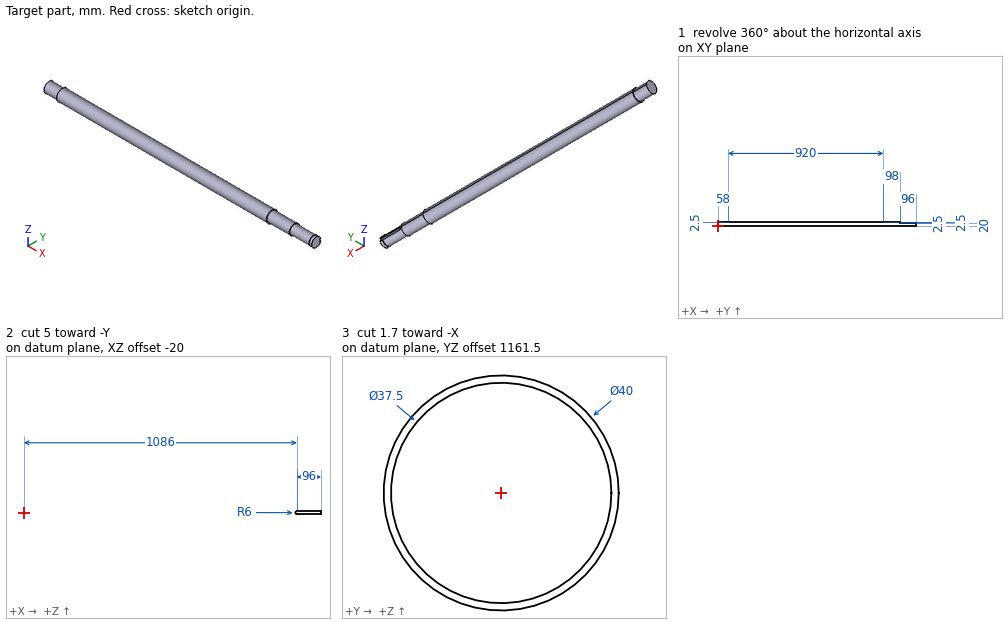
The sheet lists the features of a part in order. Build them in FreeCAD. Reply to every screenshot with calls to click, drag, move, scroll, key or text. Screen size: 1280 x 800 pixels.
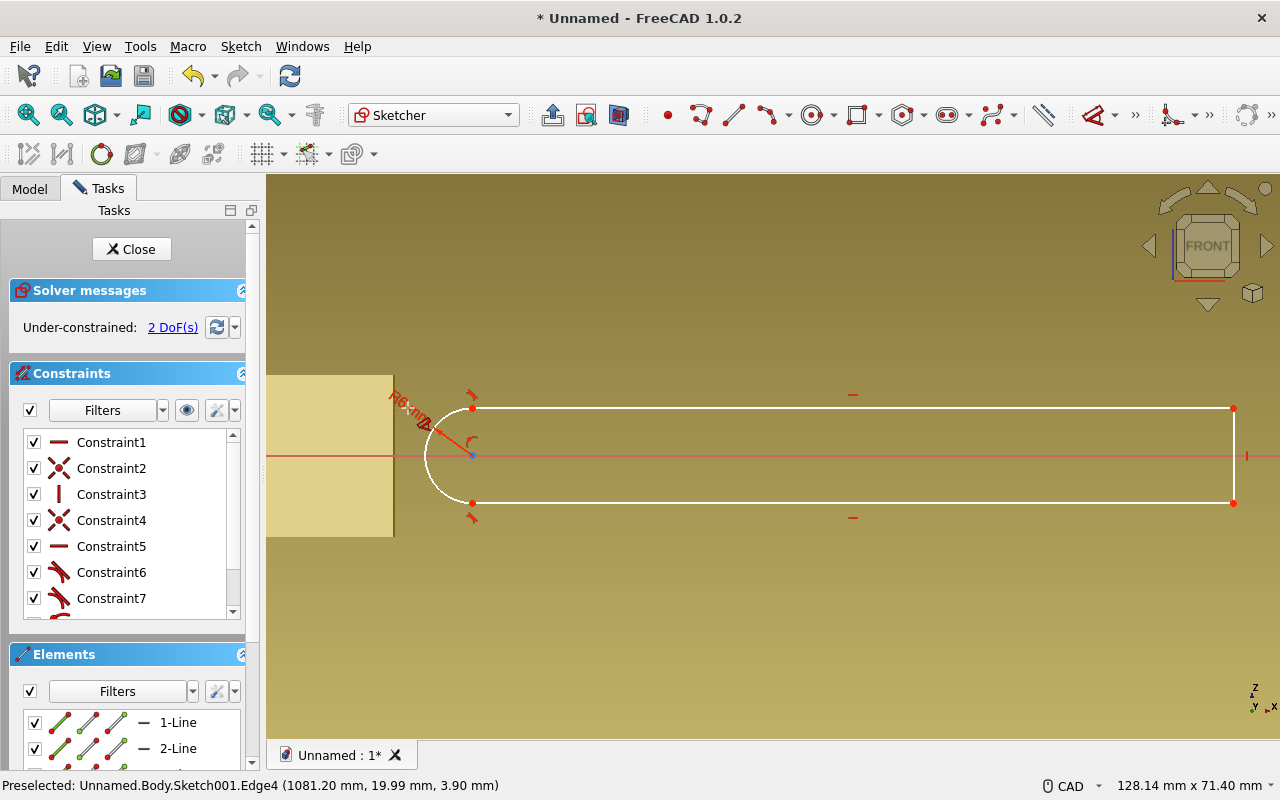
click(701, 408)
click(794, 374)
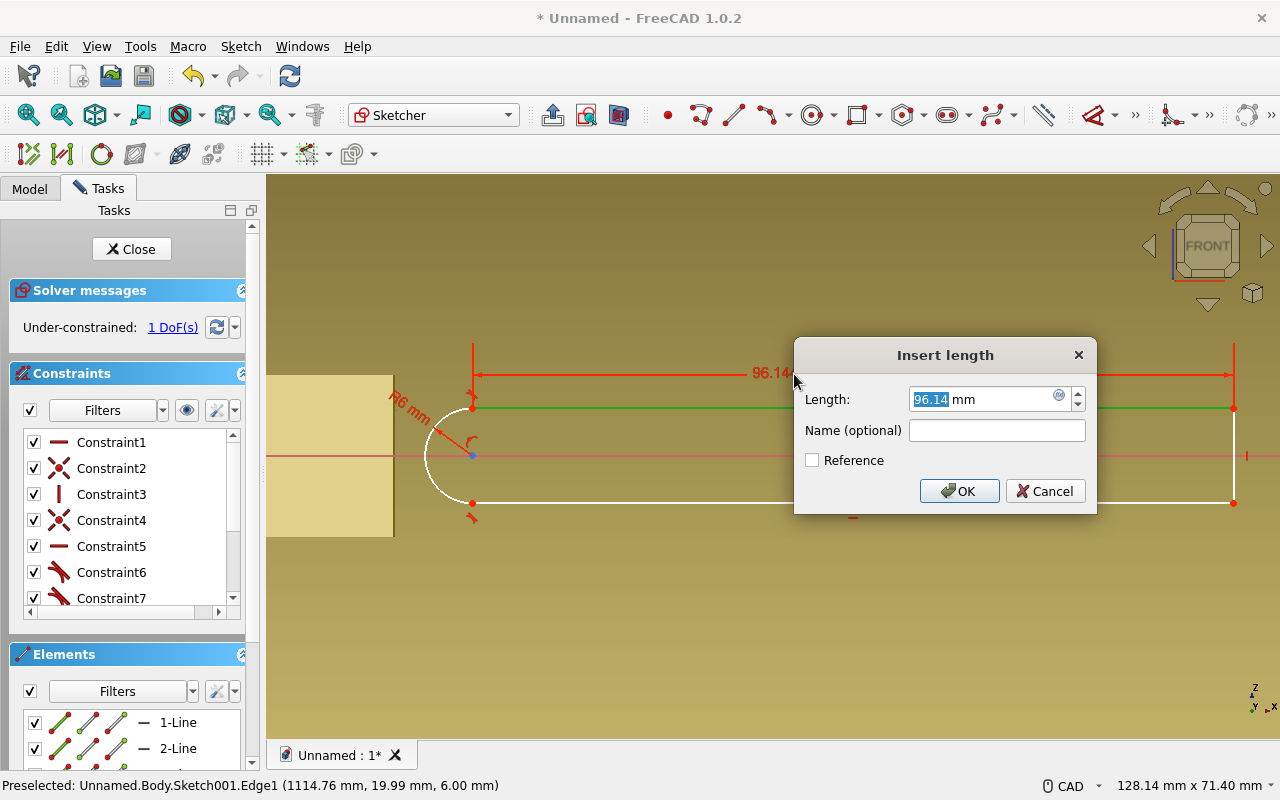
text(96)
key(Return)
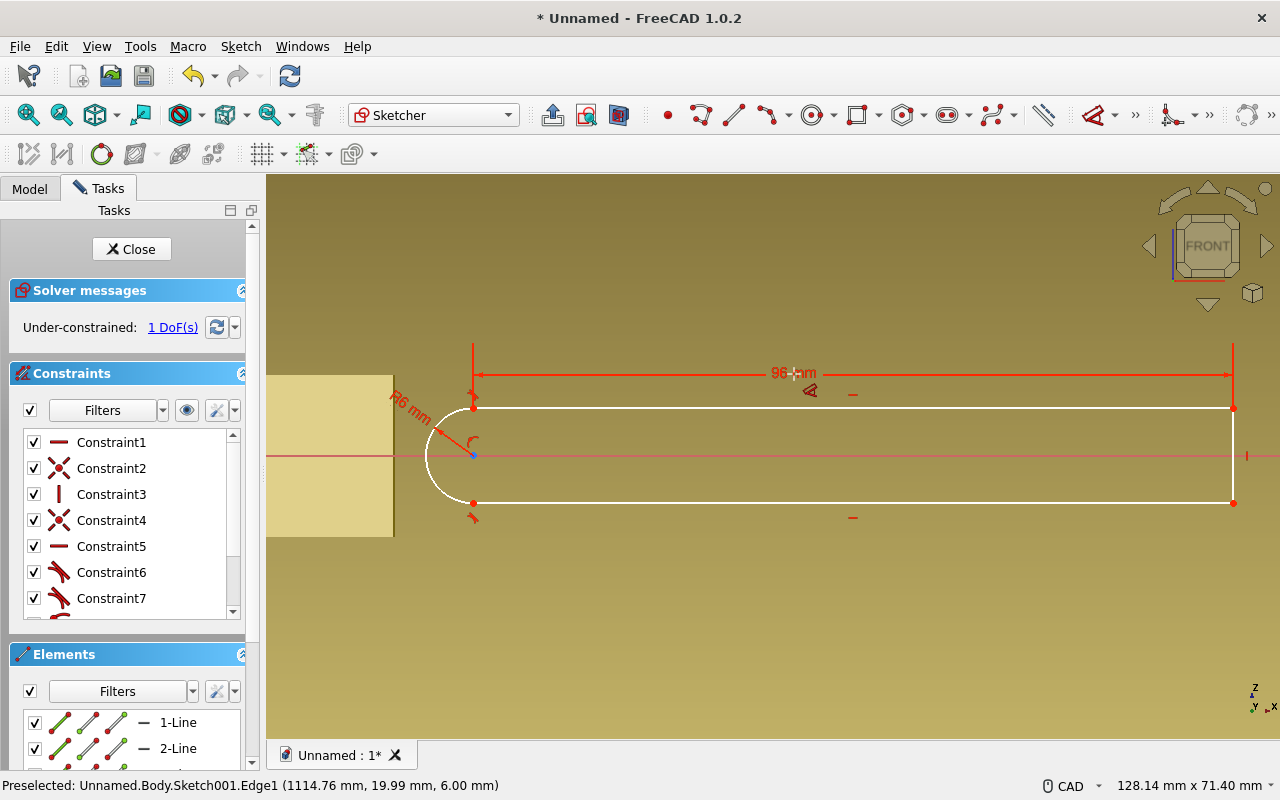
click(473, 408)
click(384, 374)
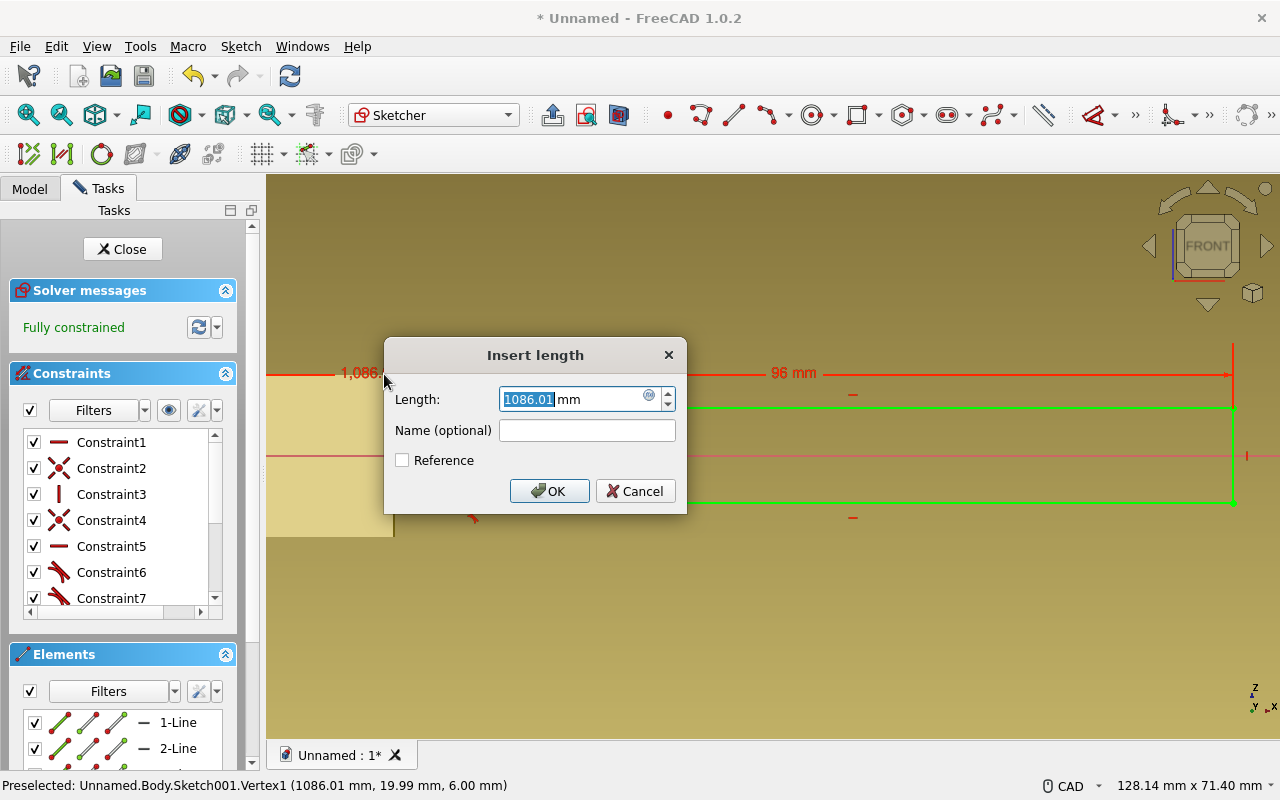
text(1086)
key(Return)
key(Escape)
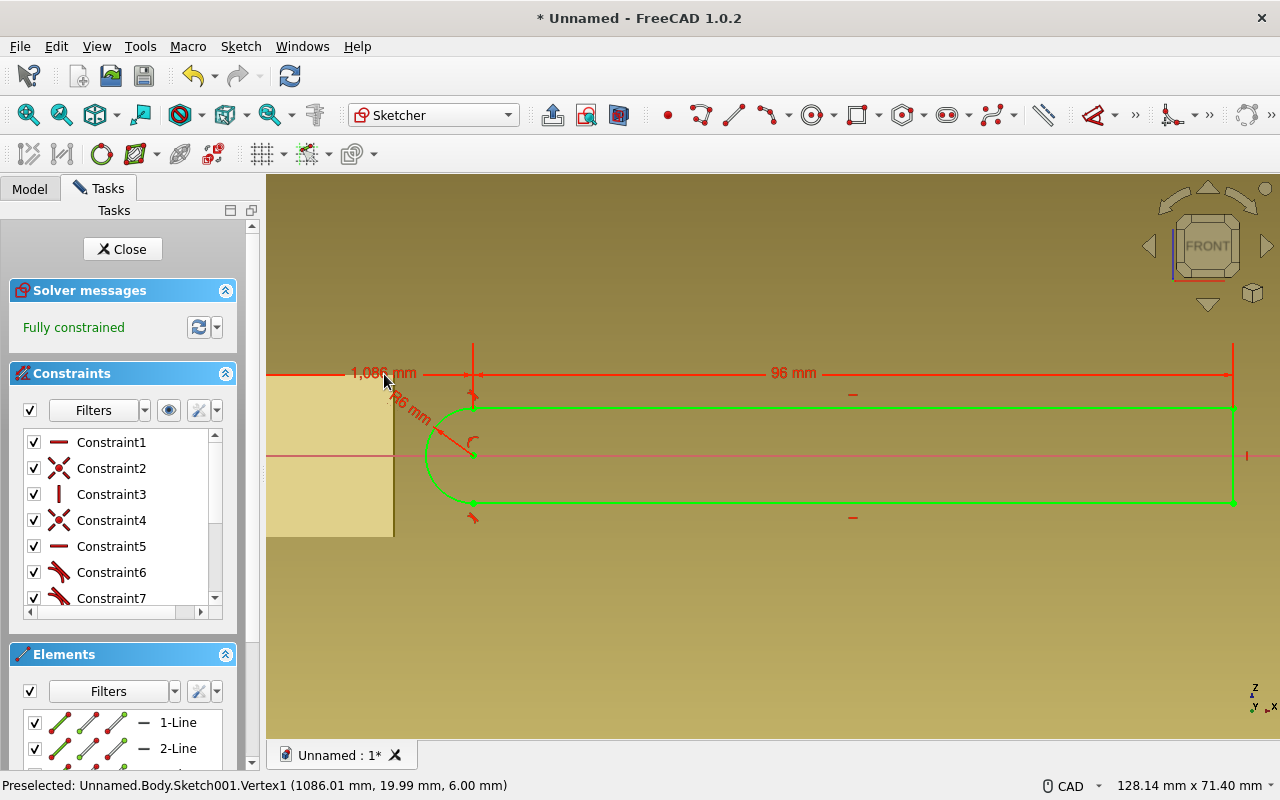
click(123, 249)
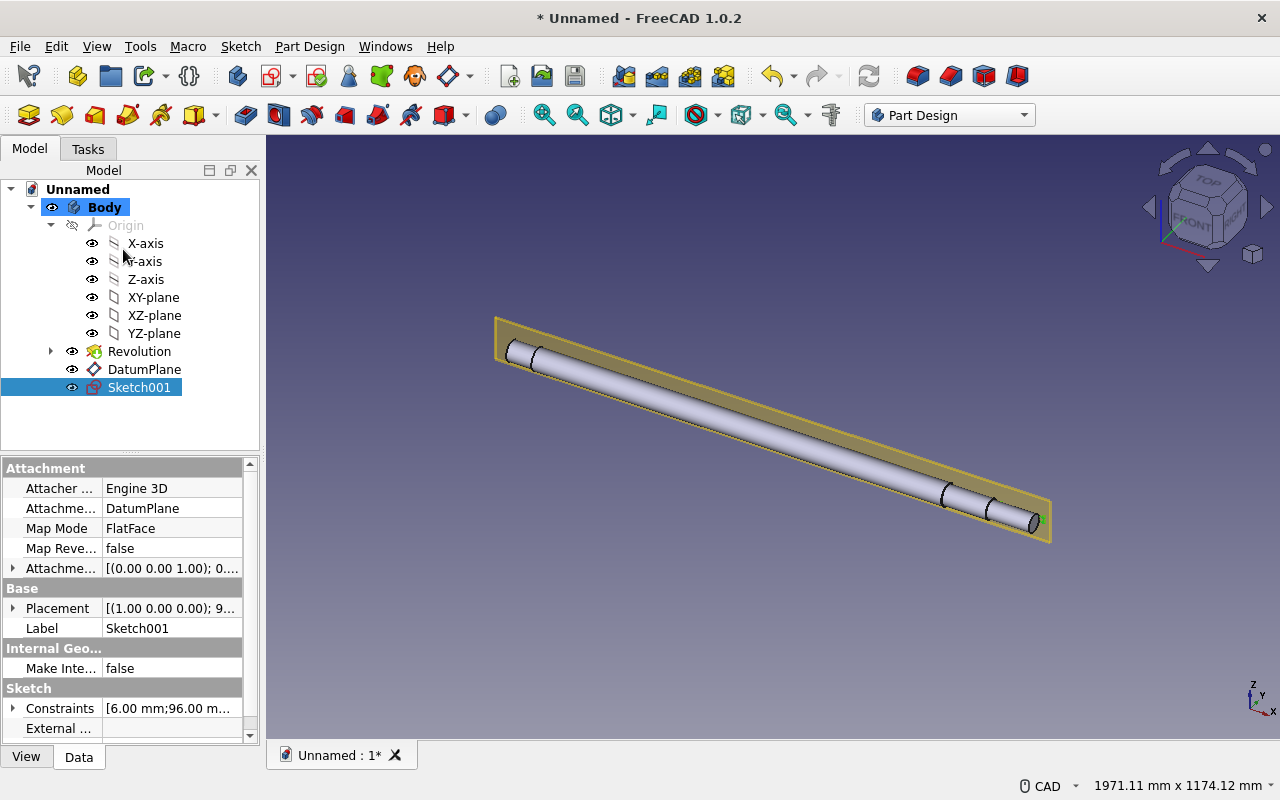
click(246, 116)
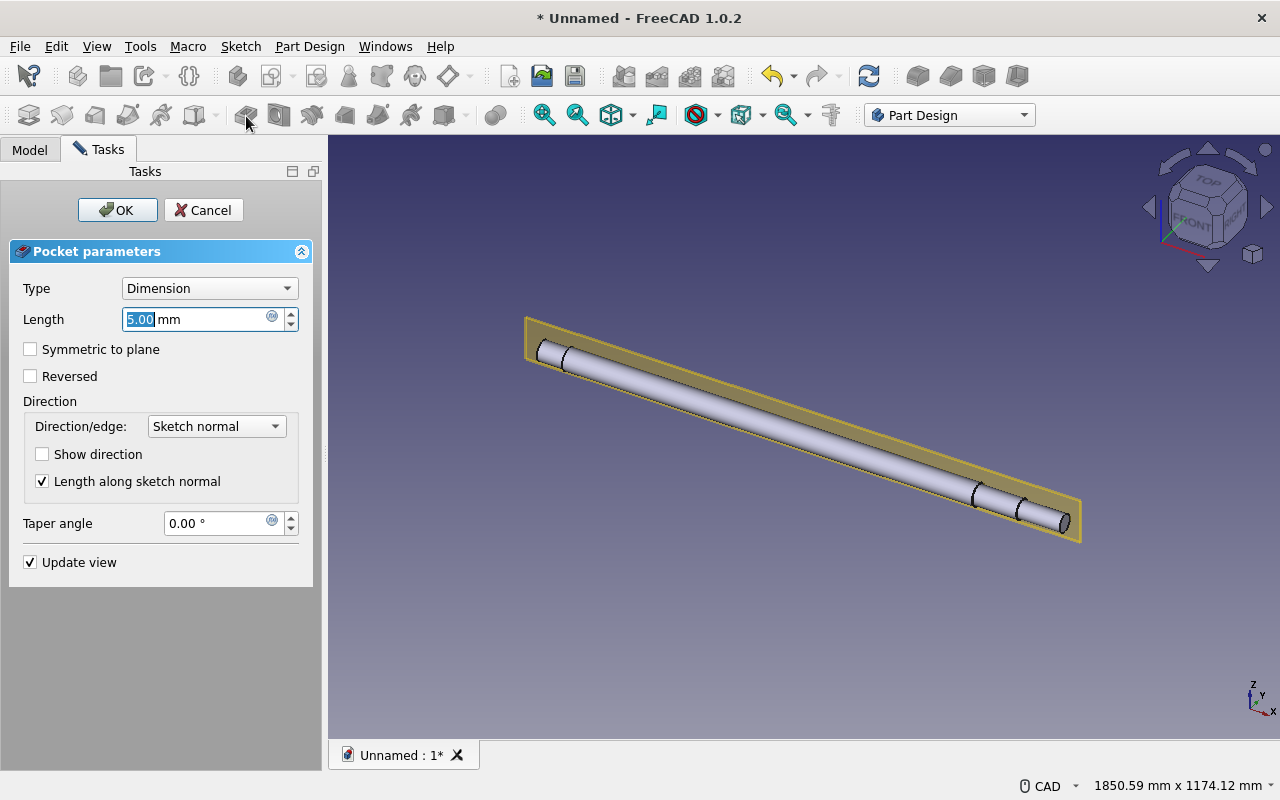
text(5)
key(Tab)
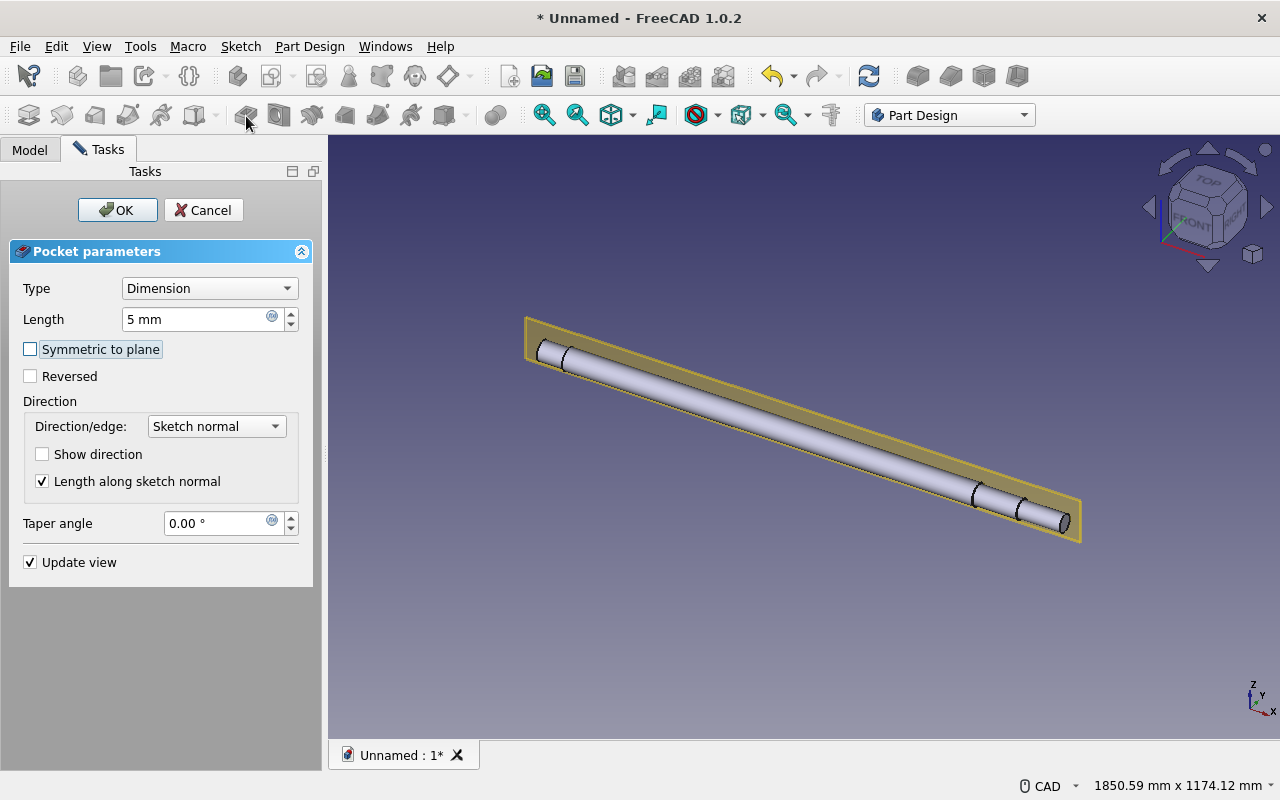
click(31, 376)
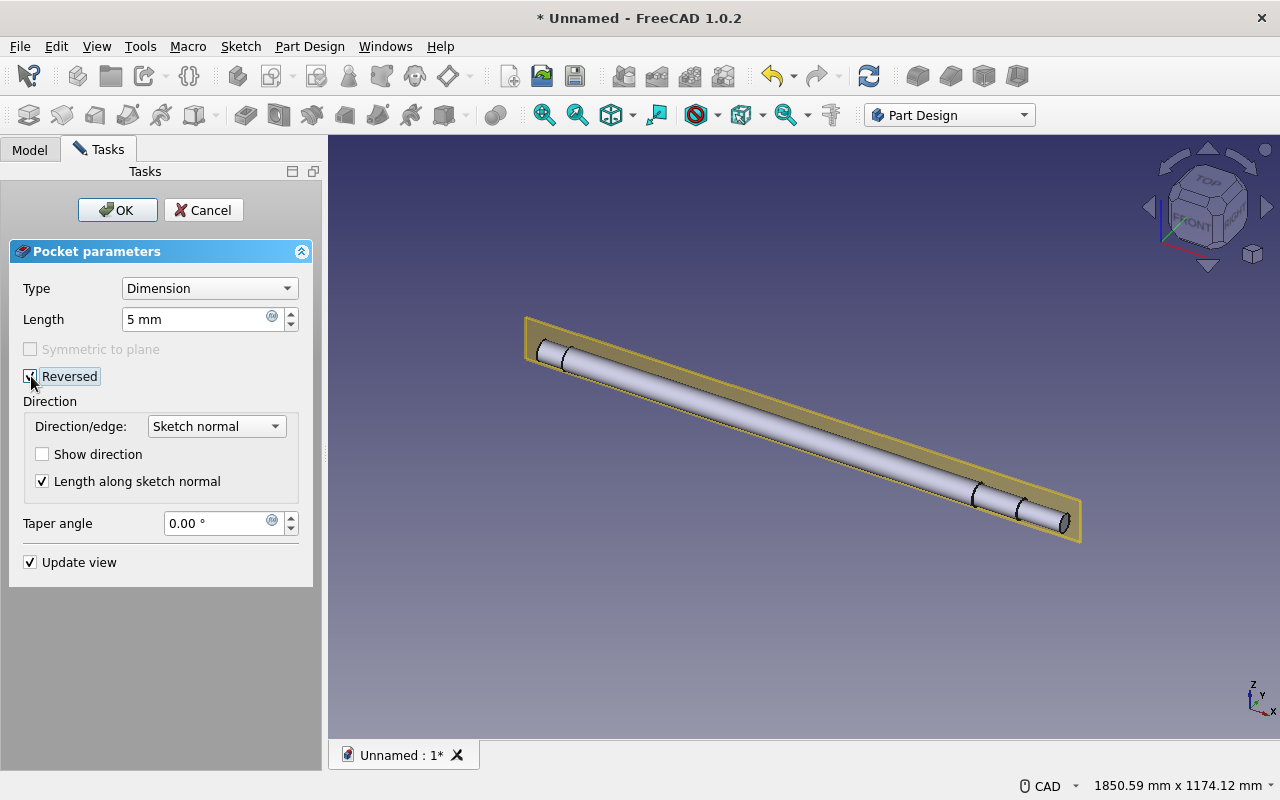
click(118, 210)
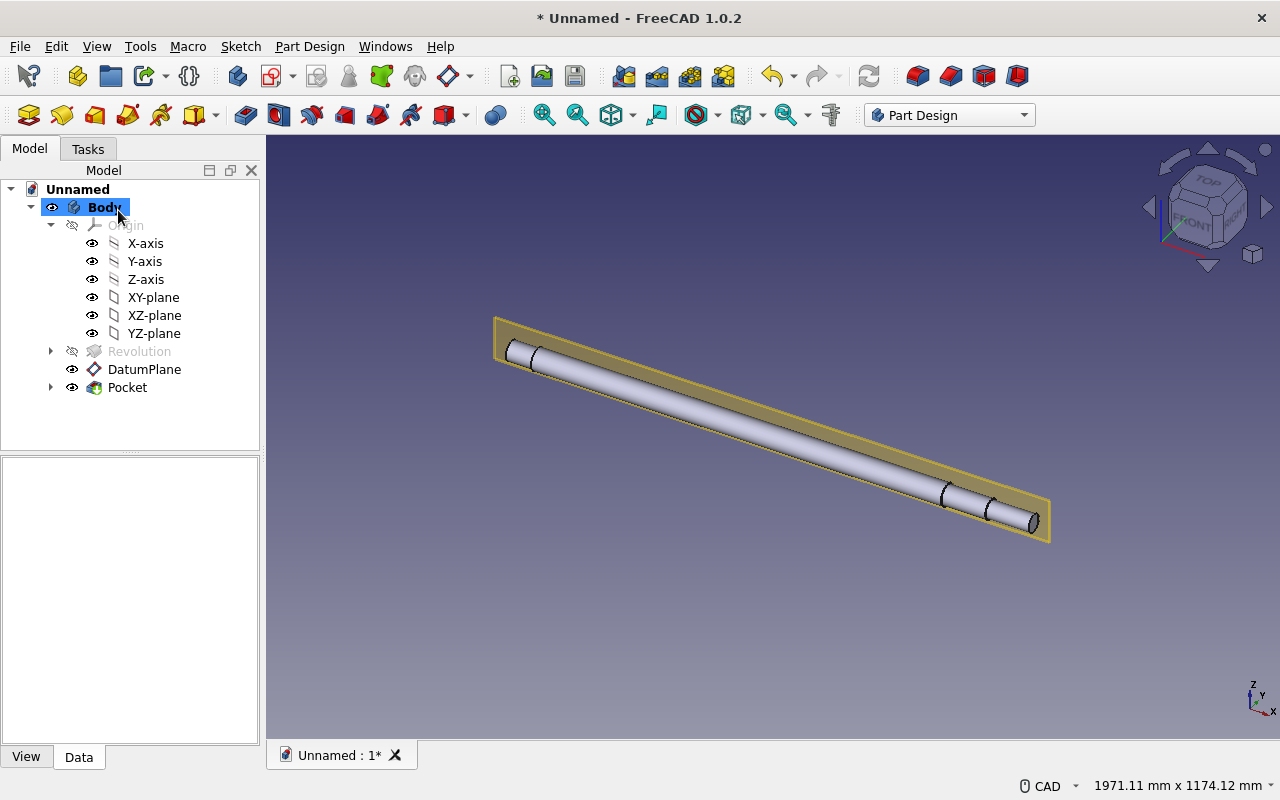
click(117, 369)
key(space)